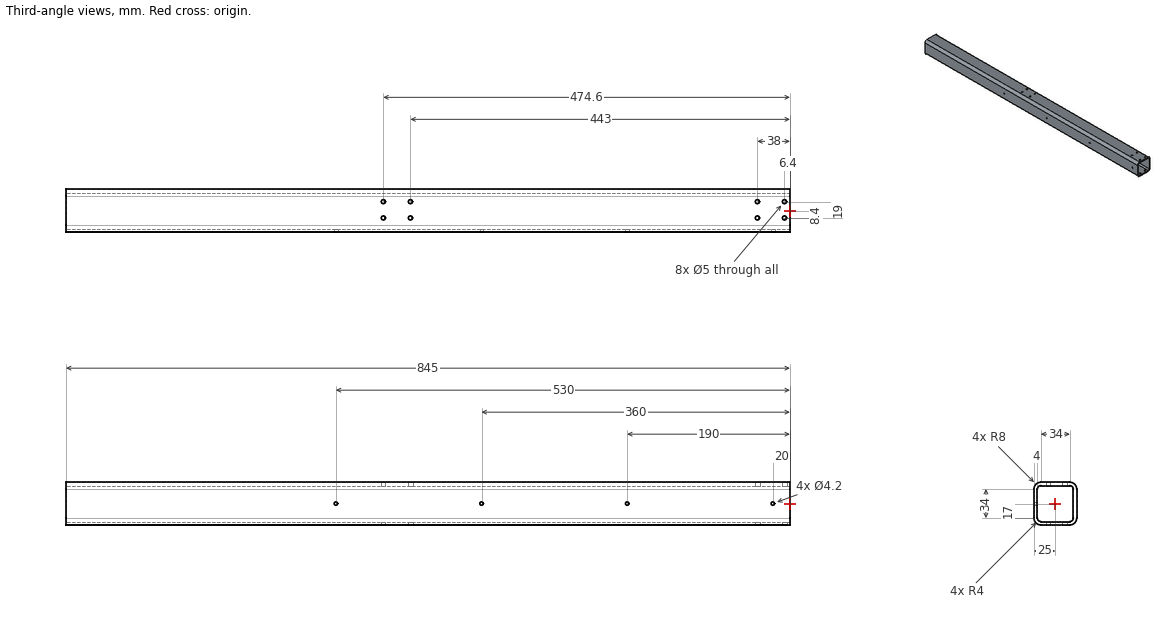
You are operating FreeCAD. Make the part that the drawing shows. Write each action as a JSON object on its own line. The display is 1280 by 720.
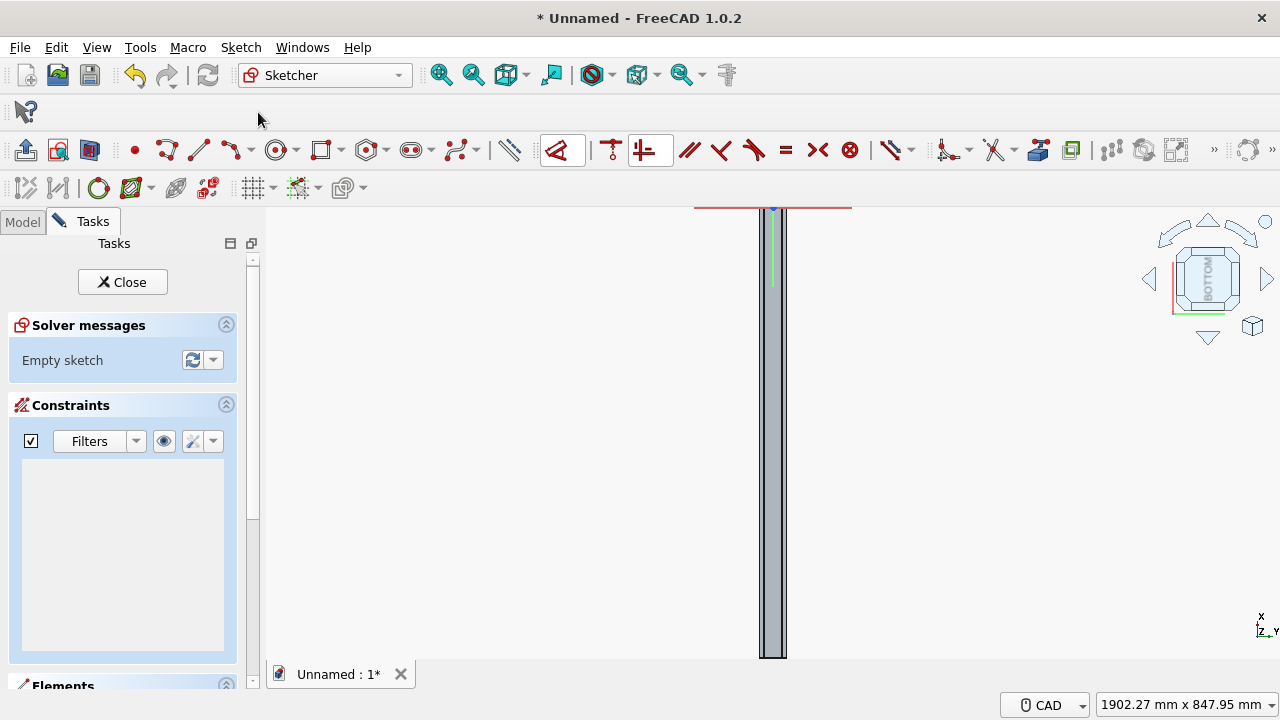
{"action": "scroll", "coordinate": [392, 631], "scroll_direction": "down", "scroll_amount": 1}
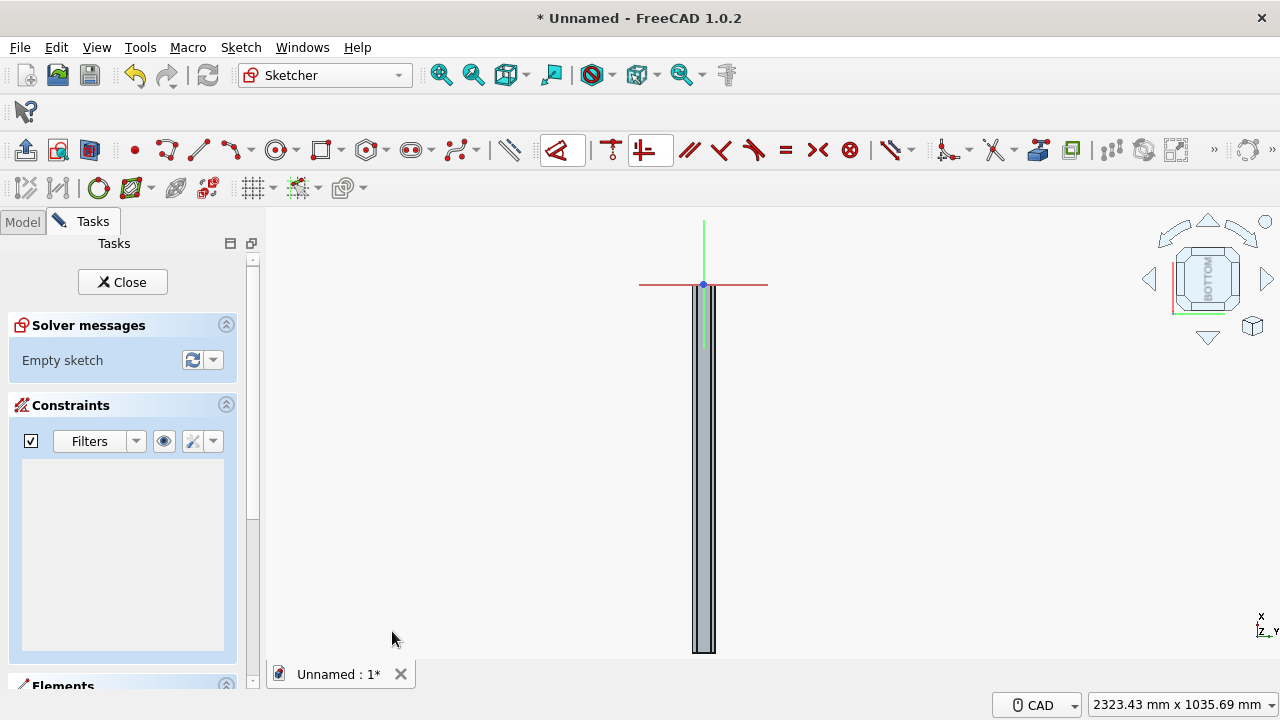
{"action": "left_click", "coordinate": [276, 150]}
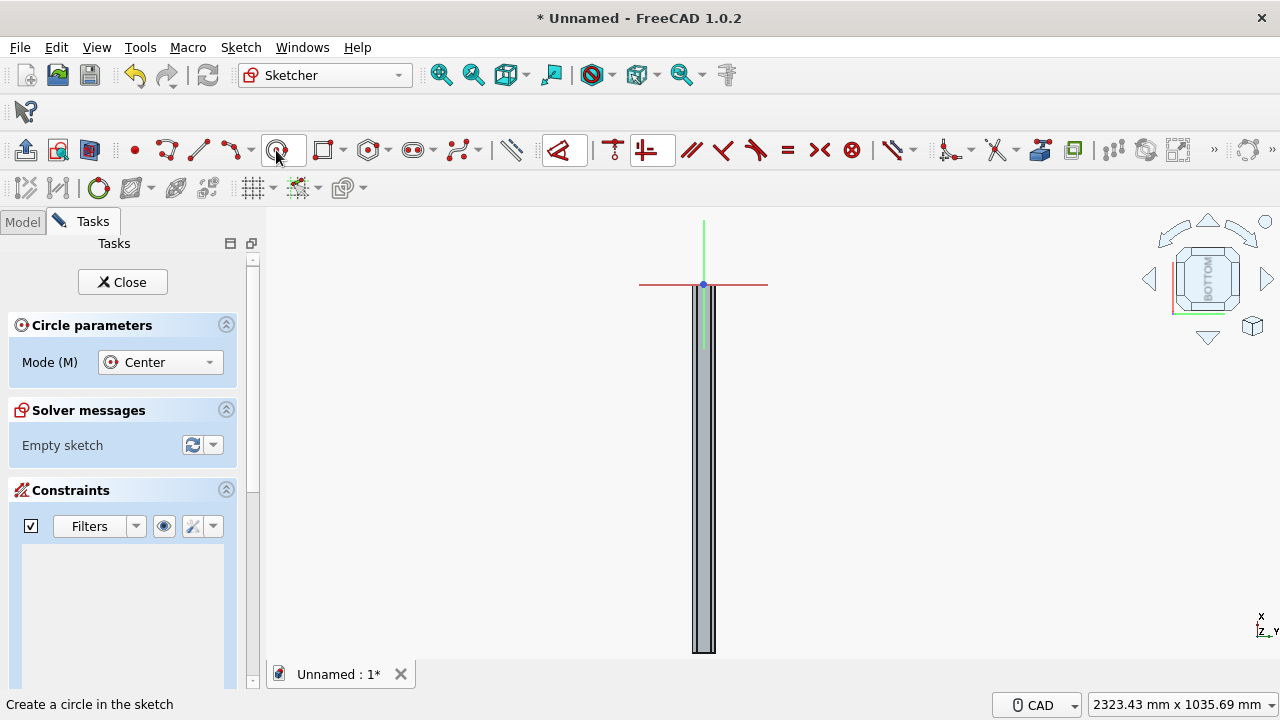
{"action": "scroll", "coordinate": [709, 287], "scroll_direction": "up", "scroll_amount": 16}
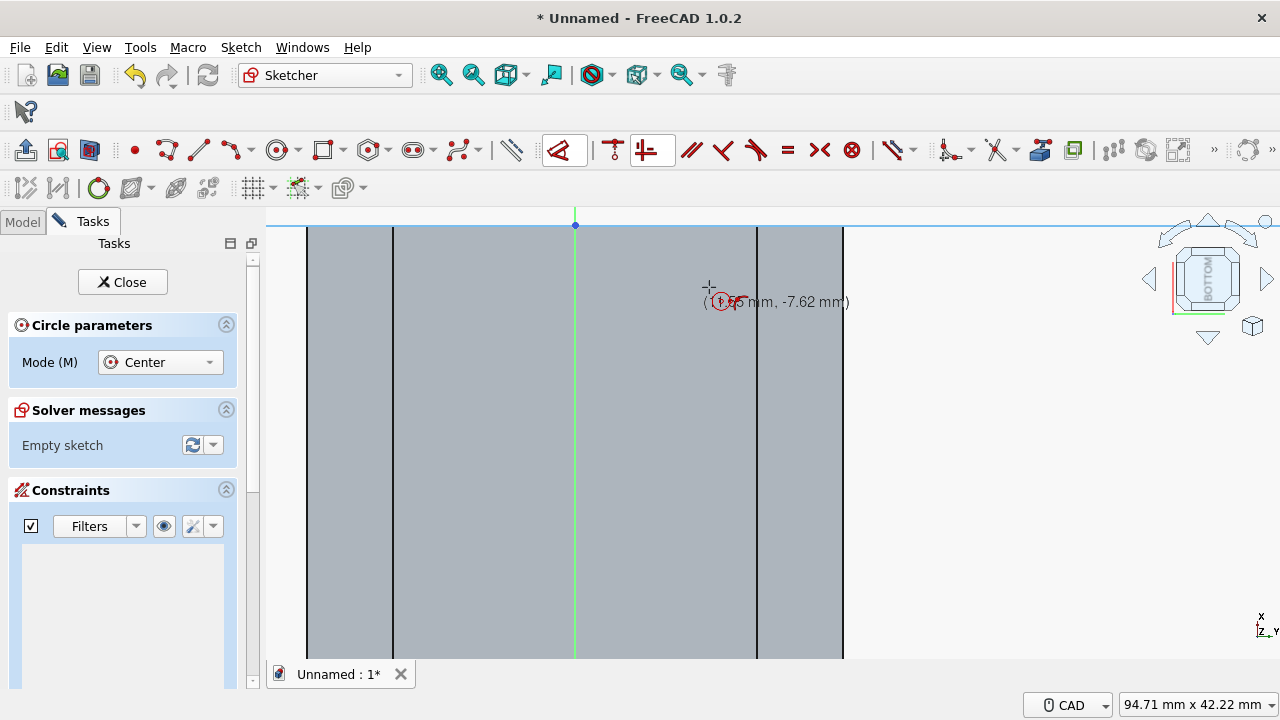
{"action": "scroll", "coordinate": [711, 310], "scroll_direction": "down", "scroll_amount": 15}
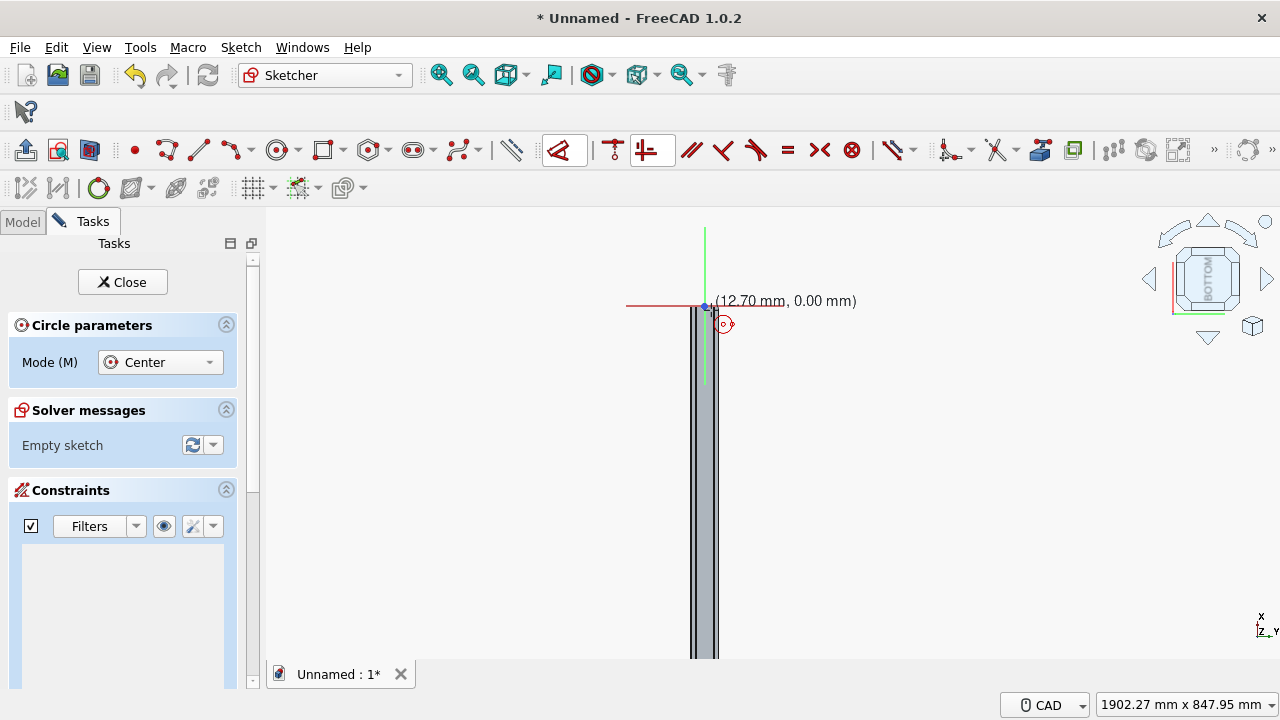
{"action": "scroll", "coordinate": [710, 309], "scroll_direction": "up", "scroll_amount": 8}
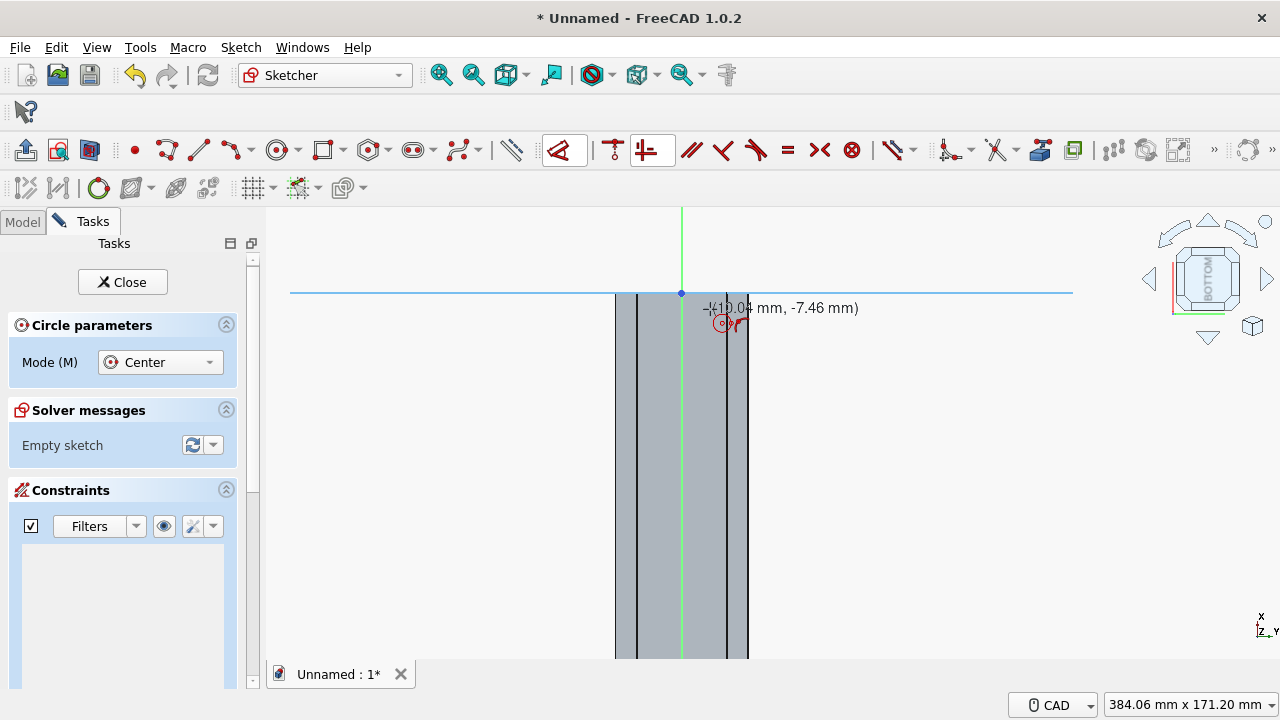
{"action": "left_click", "coordinate": [710, 310]}
{"action": "mouse_move", "coordinate": [714, 315]}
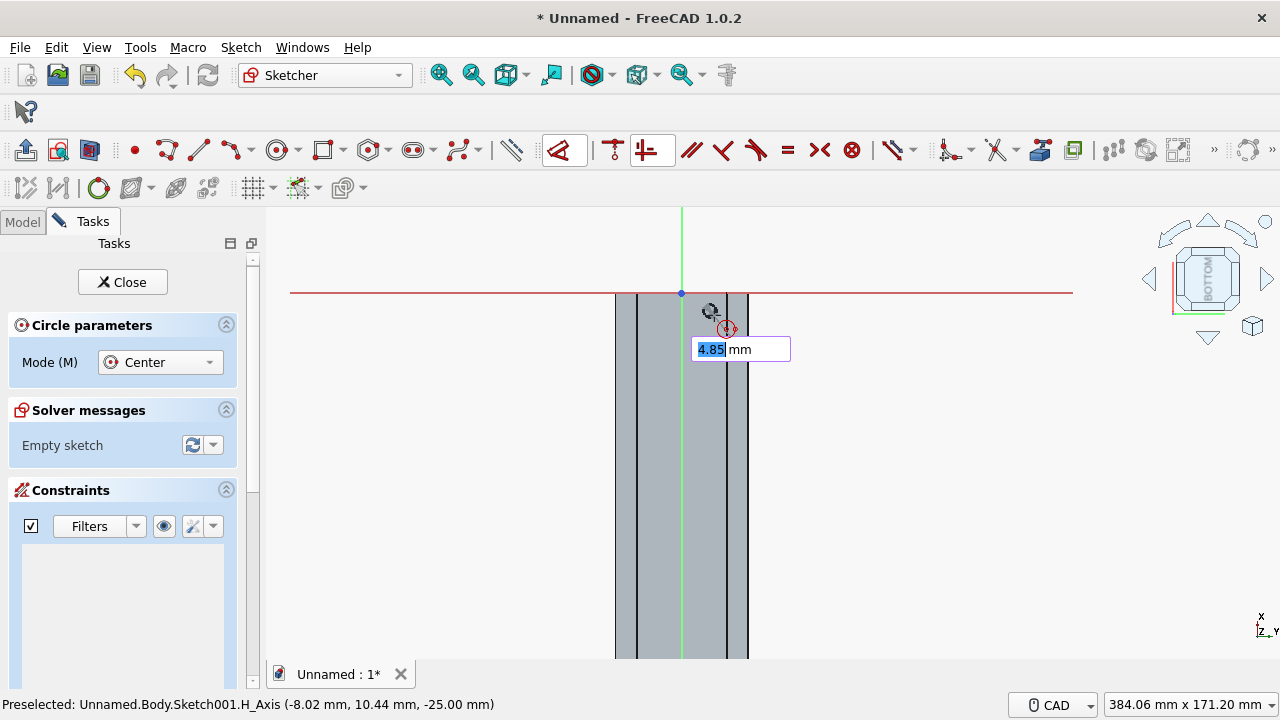
{"action": "type", "text": "5"}
{"action": "key", "text": "Return"}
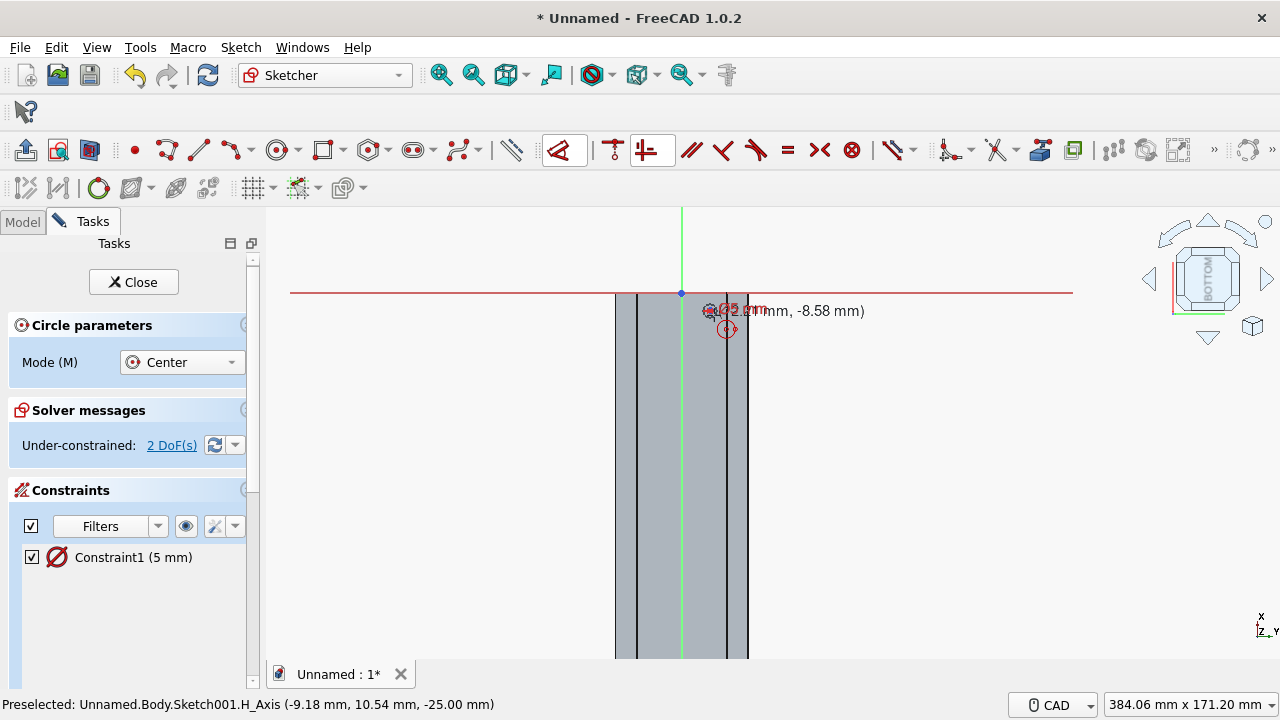
{"action": "scroll", "coordinate": [660, 310], "scroll_direction": "up", "scroll_amount": 7}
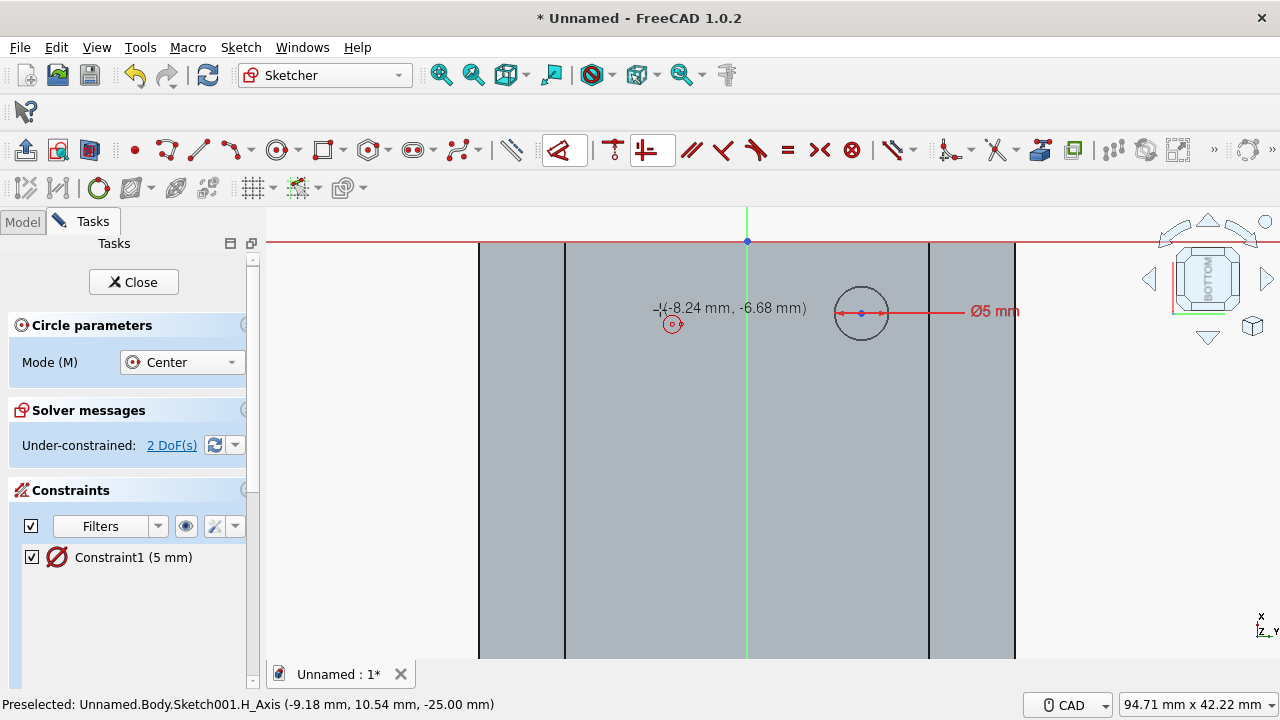
{"action": "scroll", "coordinate": [702, 309], "scroll_direction": "down", "scroll_amount": 15}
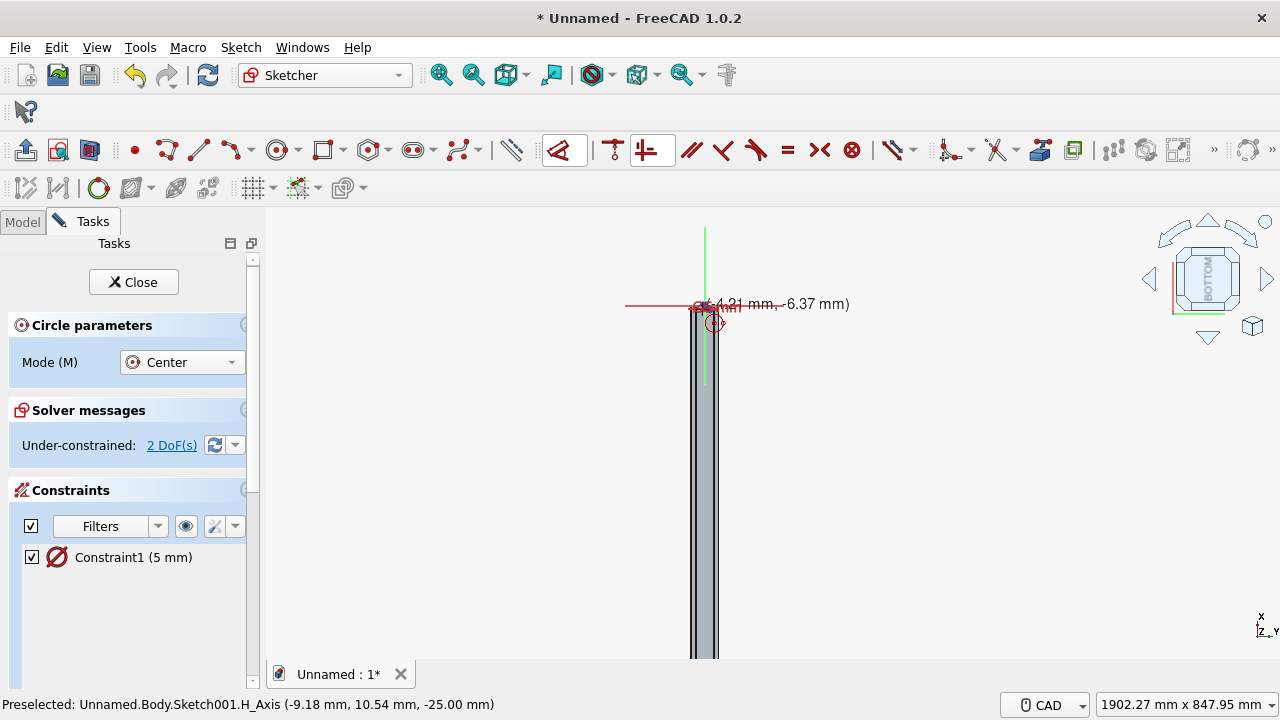
{"action": "scroll", "coordinate": [700, 309], "scroll_direction": "up", "scroll_amount": 8}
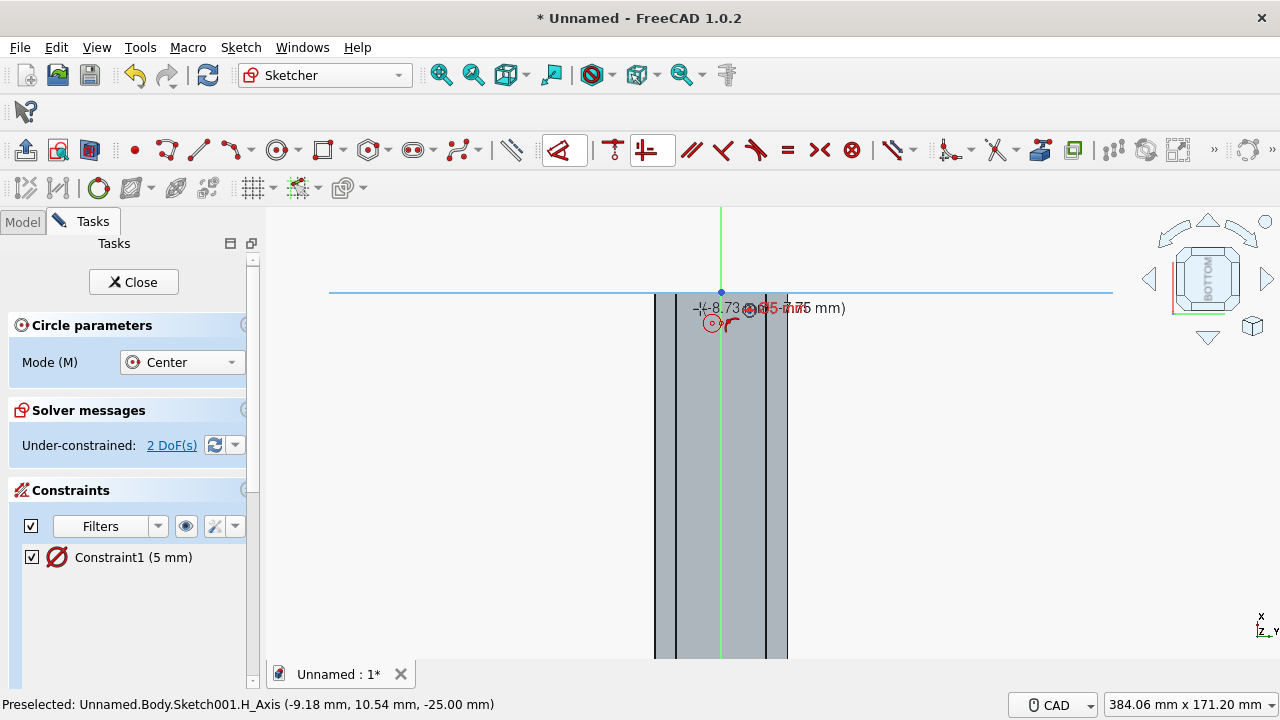
{"action": "left_click", "coordinate": [699, 309]}
{"action": "mouse_move", "coordinate": [704, 314]}